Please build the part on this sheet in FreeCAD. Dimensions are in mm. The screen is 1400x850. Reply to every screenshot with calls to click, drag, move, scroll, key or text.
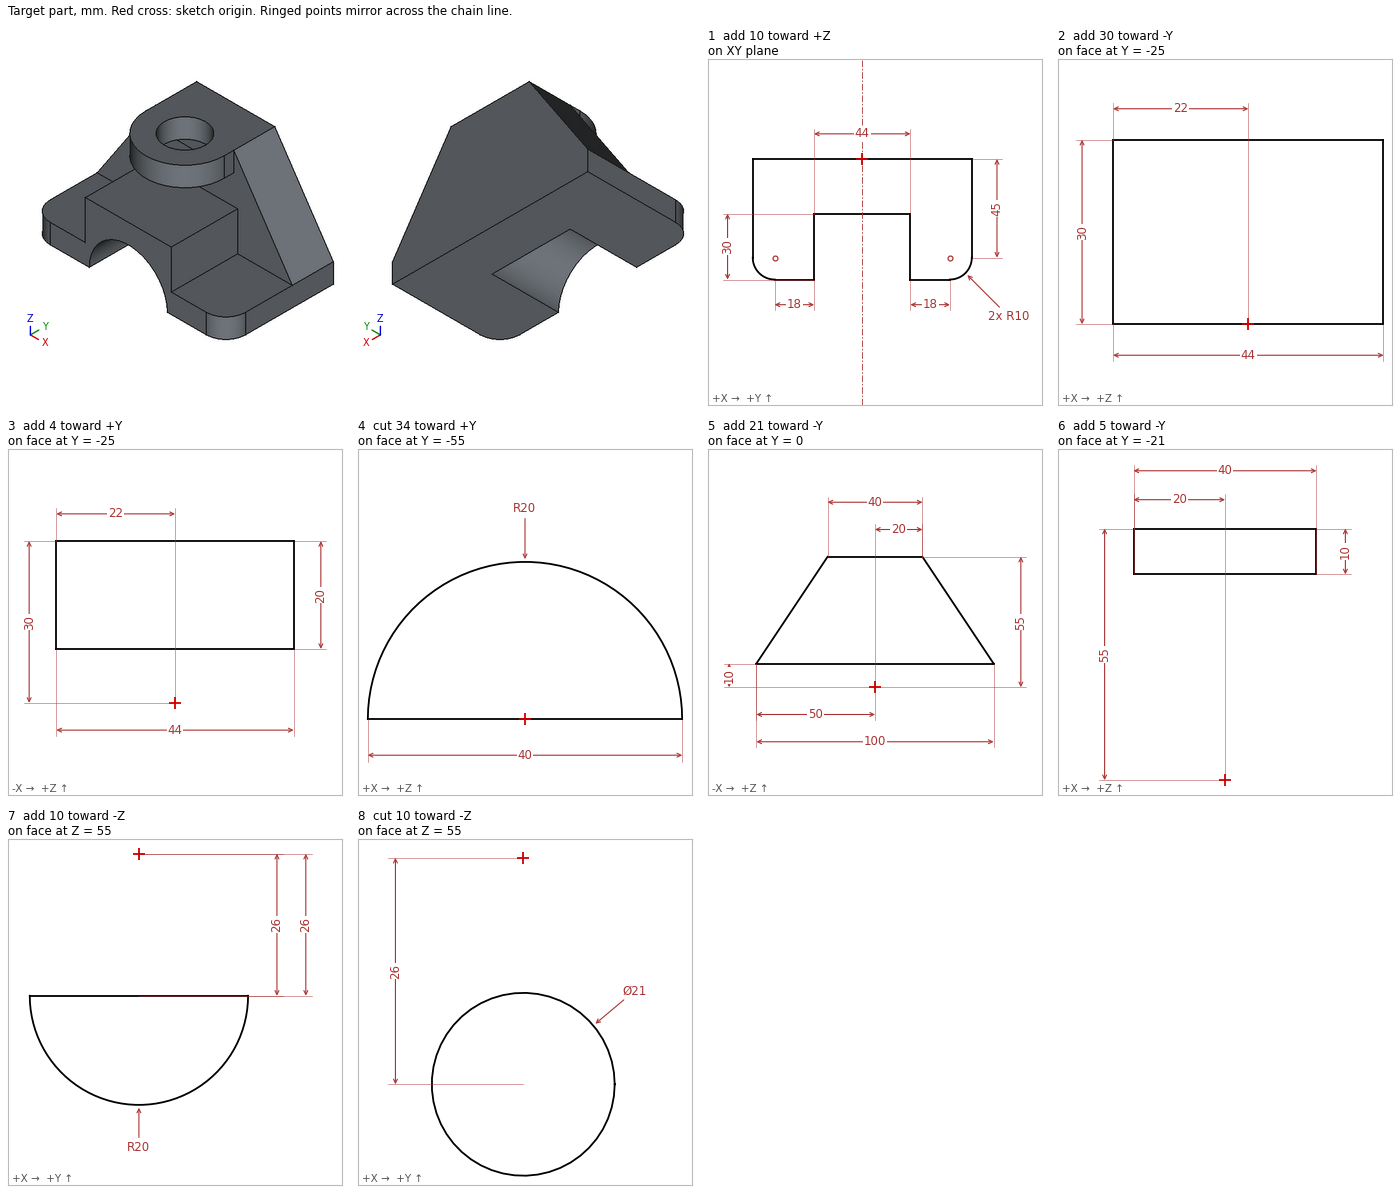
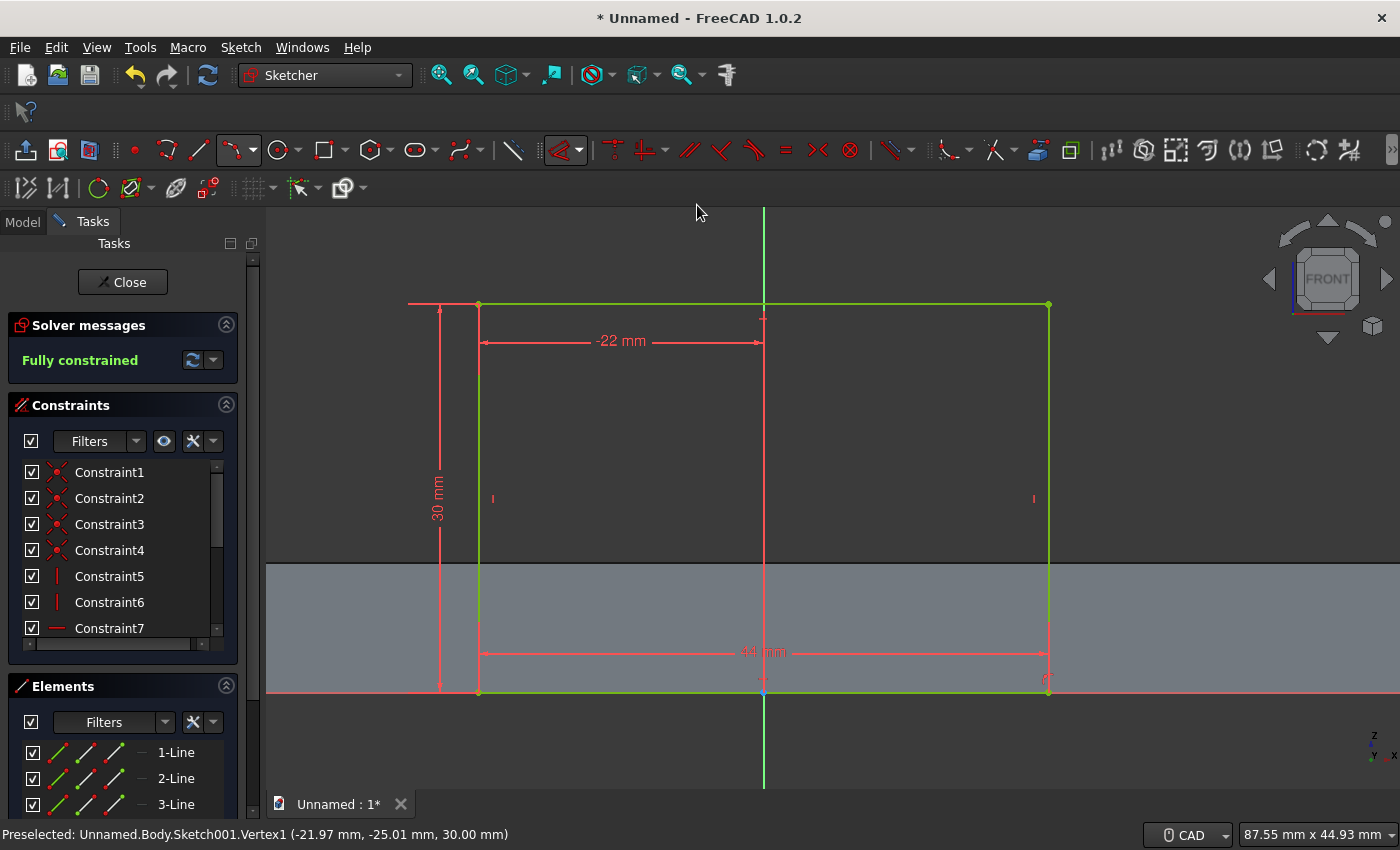
click(123, 282)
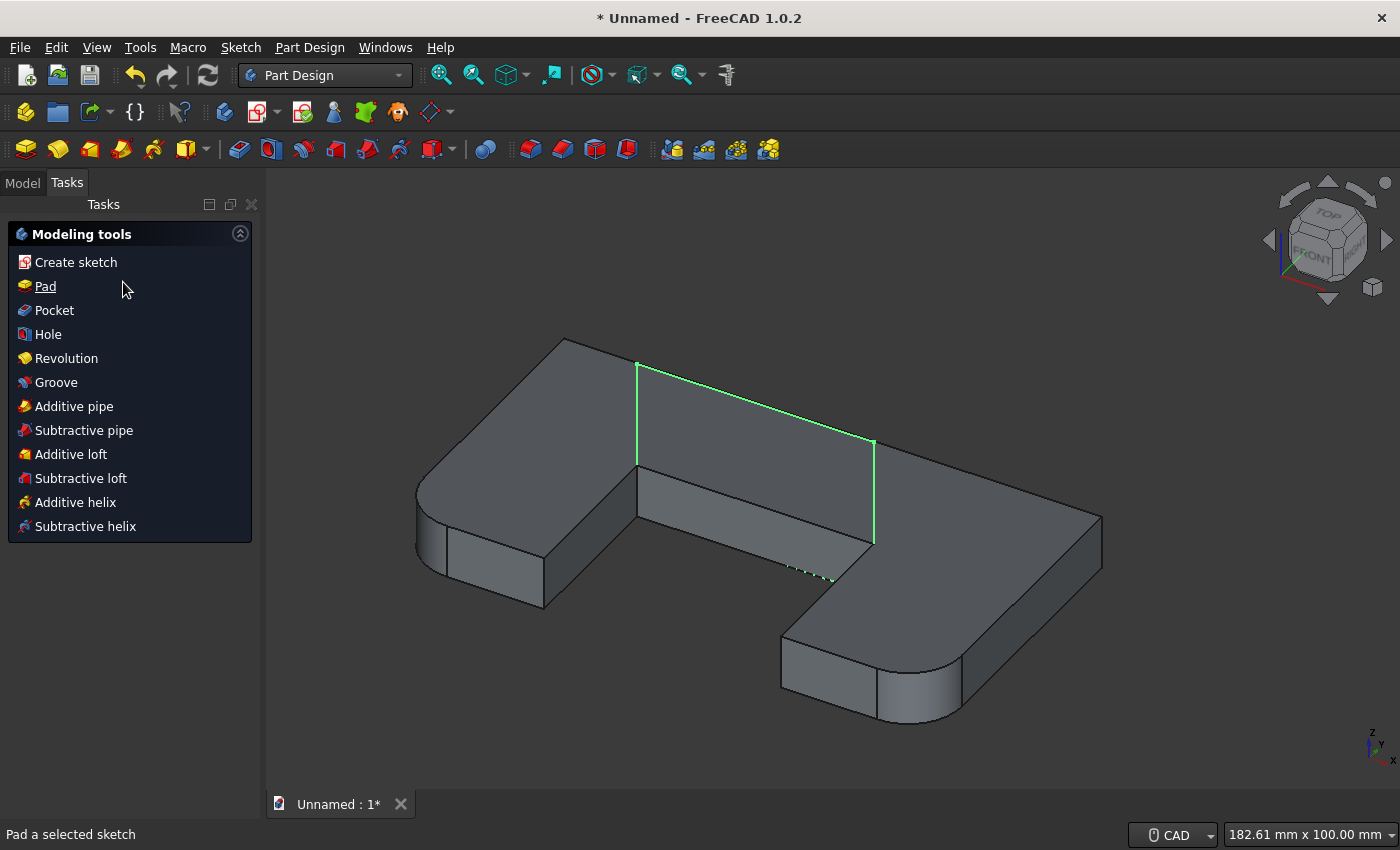
click(26, 150)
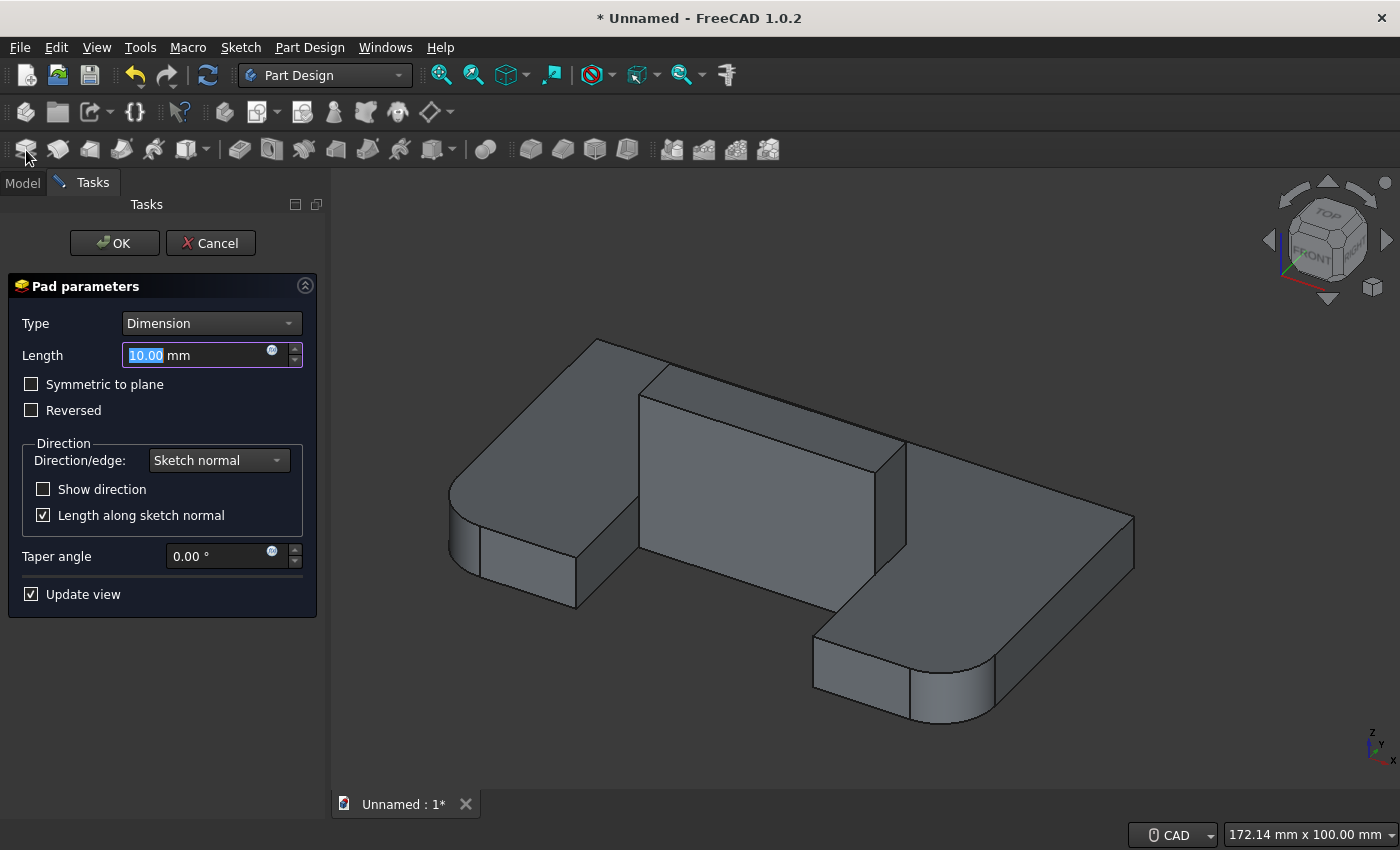
text(30)
key(Tab)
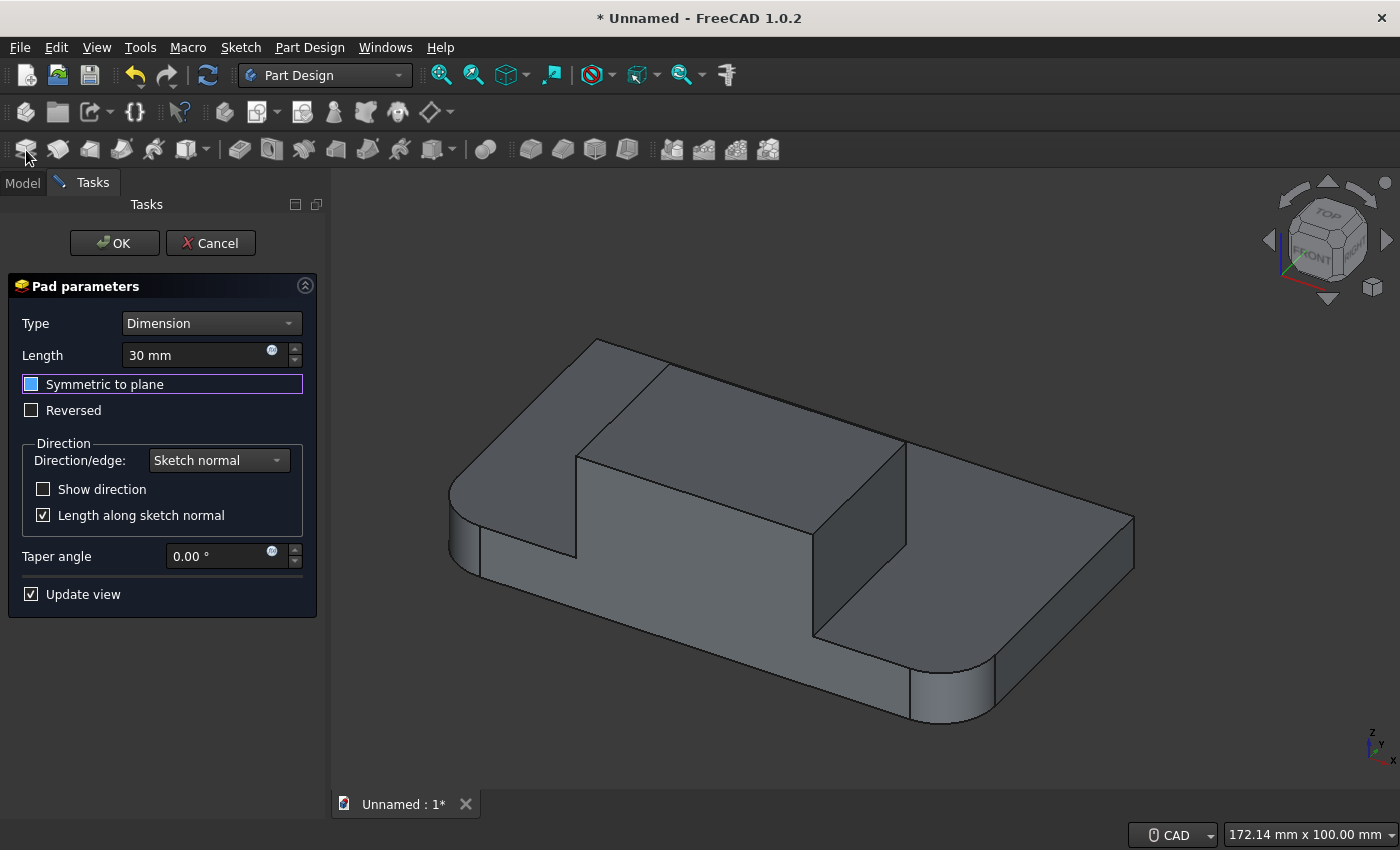
click(115, 243)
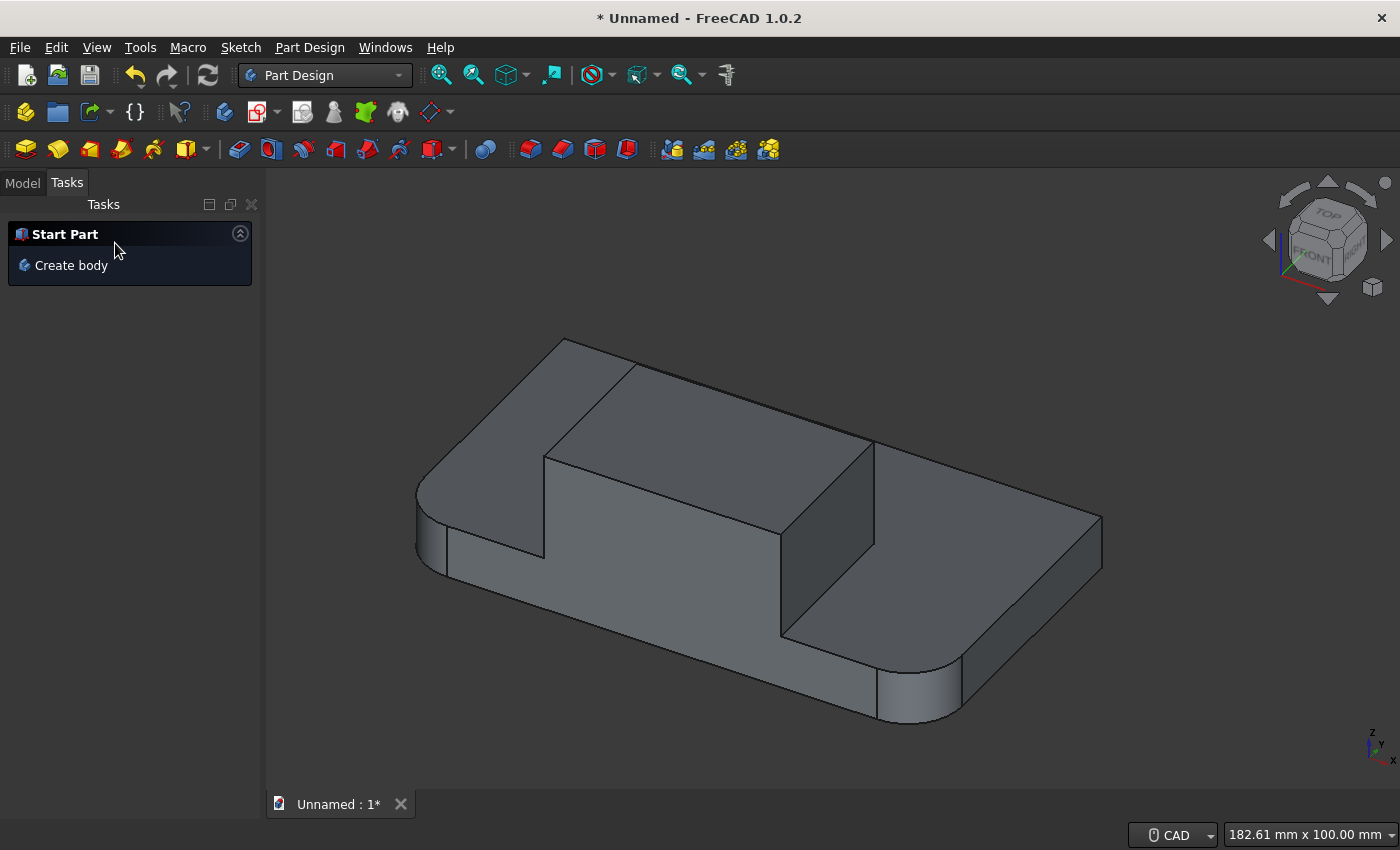
key(4)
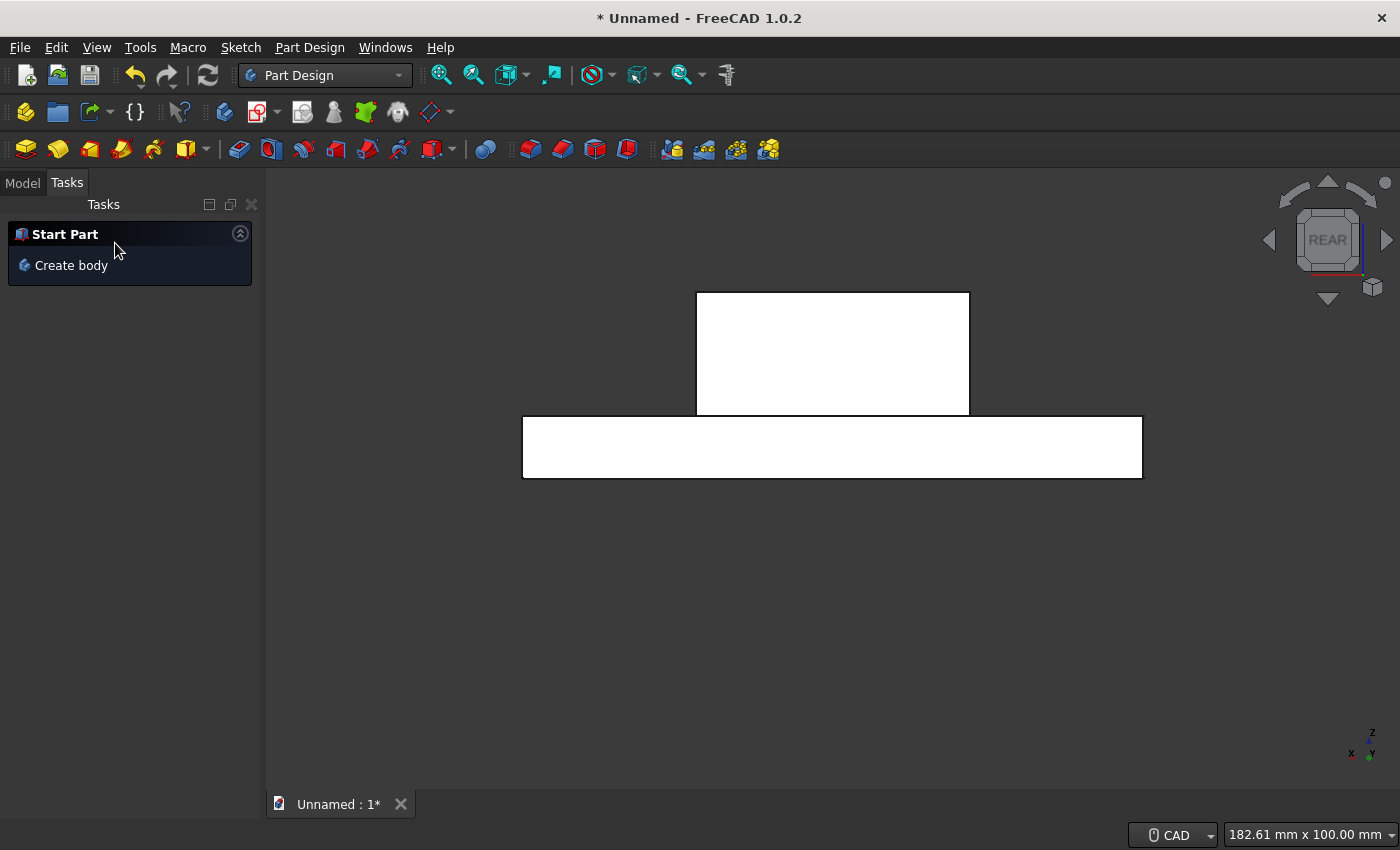
click(794, 353)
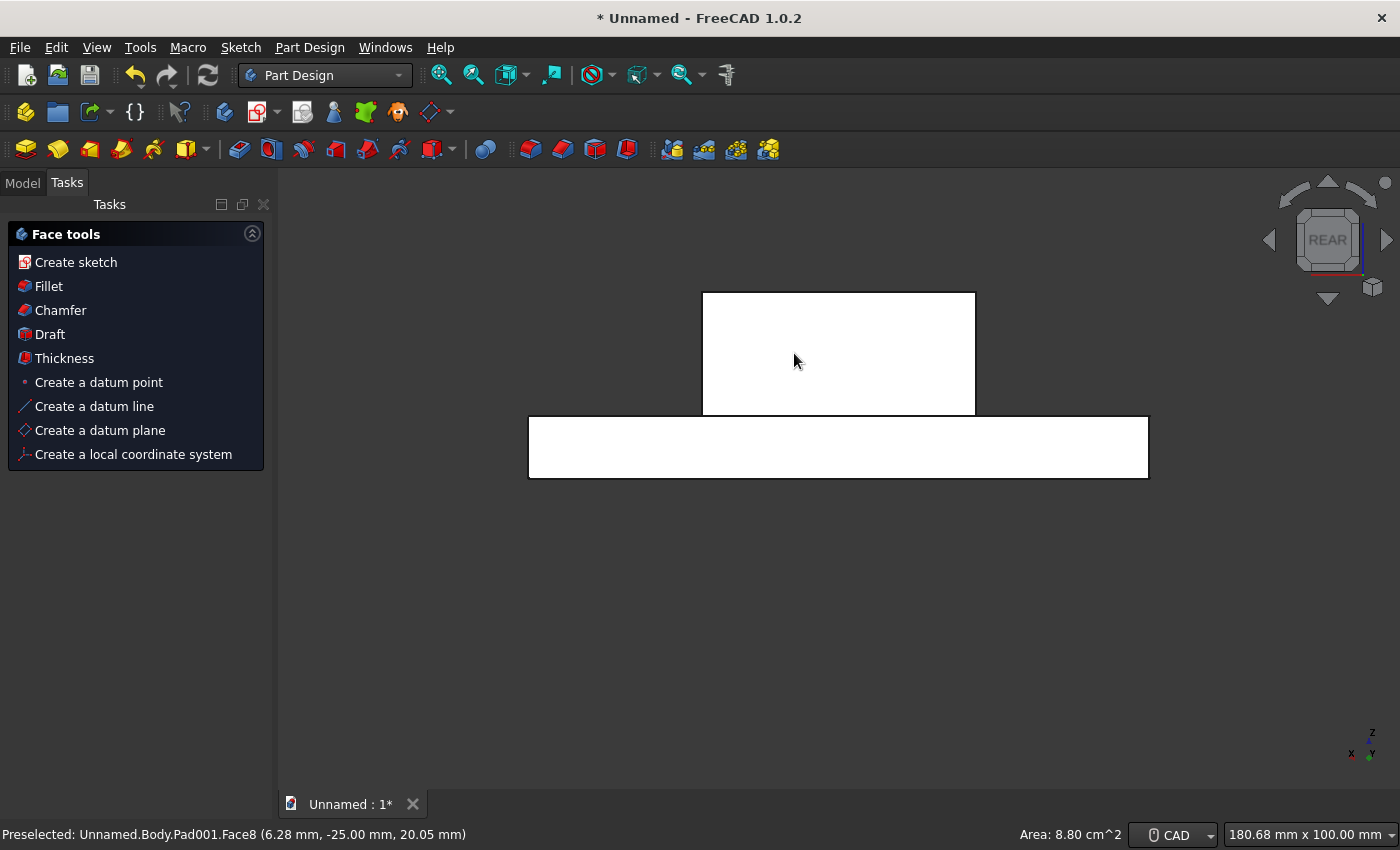
click(258, 112)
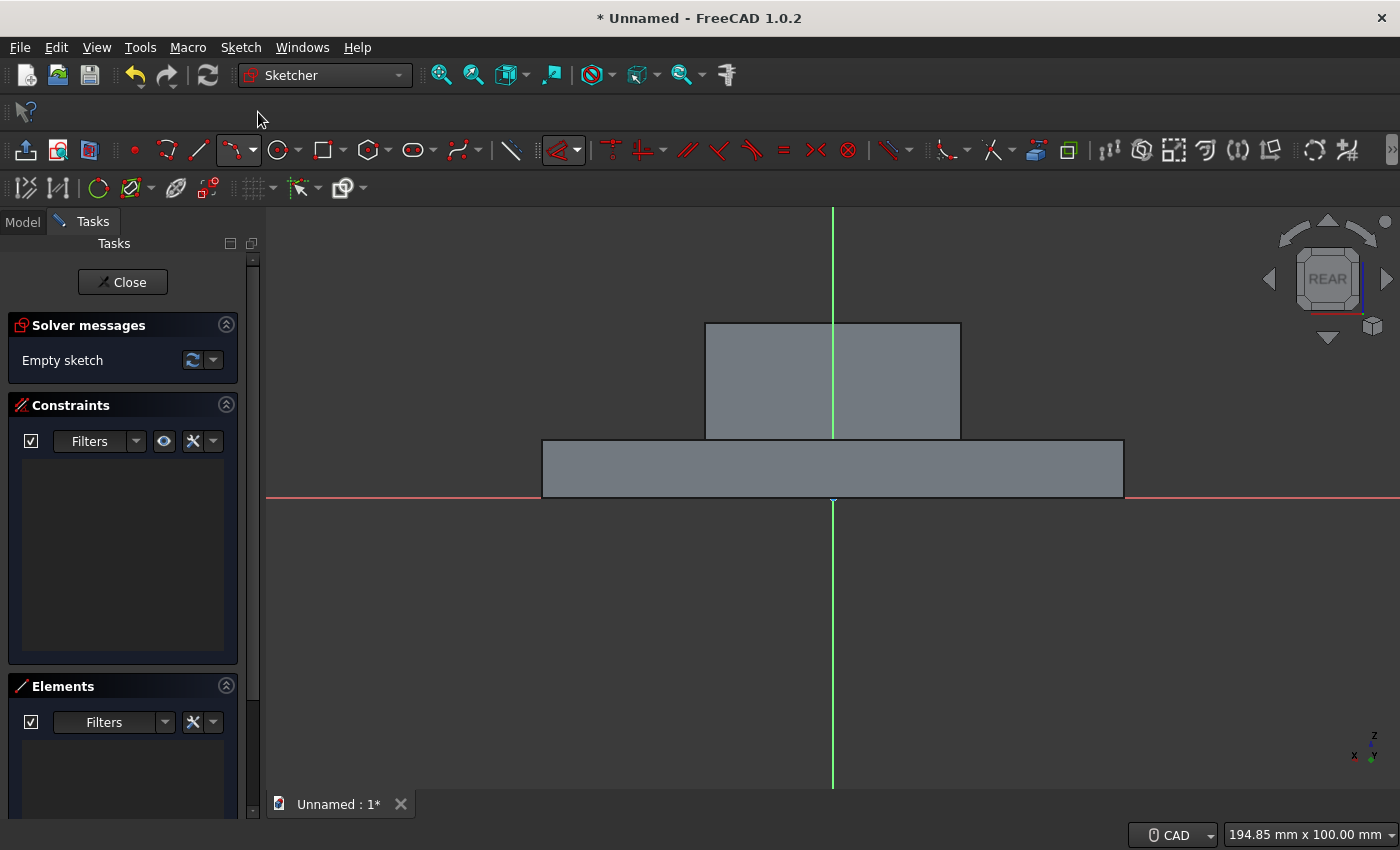
scroll(889, 339, up, 4)